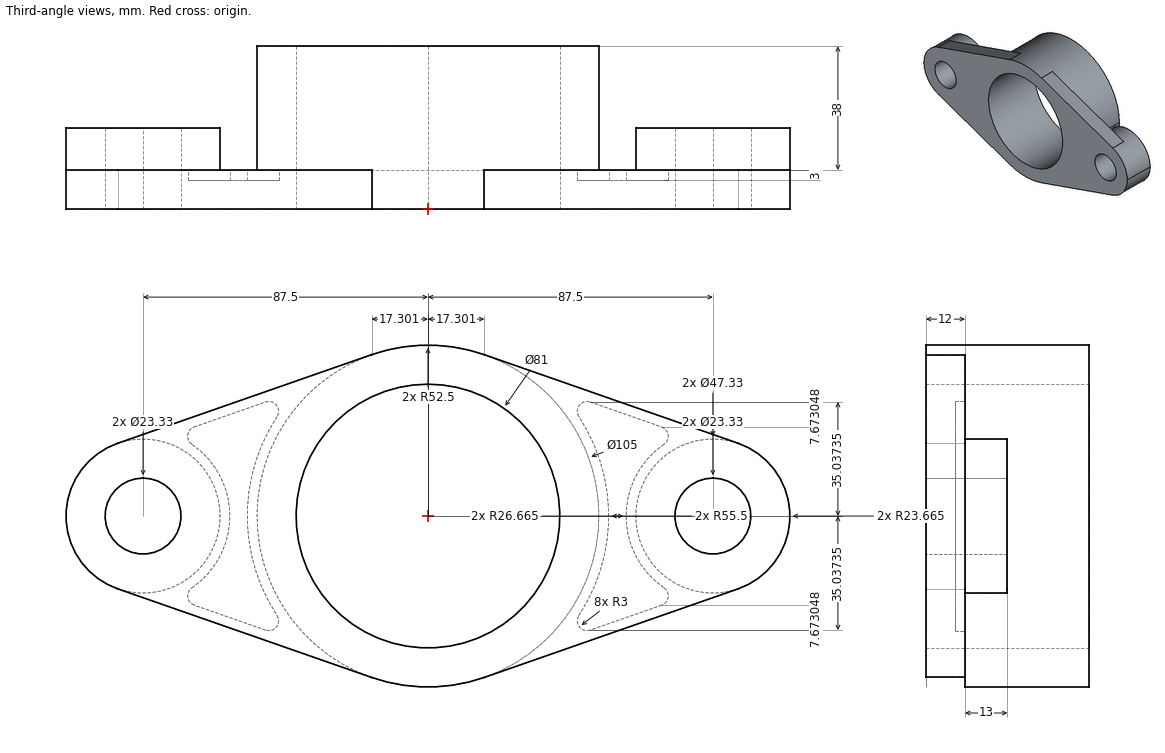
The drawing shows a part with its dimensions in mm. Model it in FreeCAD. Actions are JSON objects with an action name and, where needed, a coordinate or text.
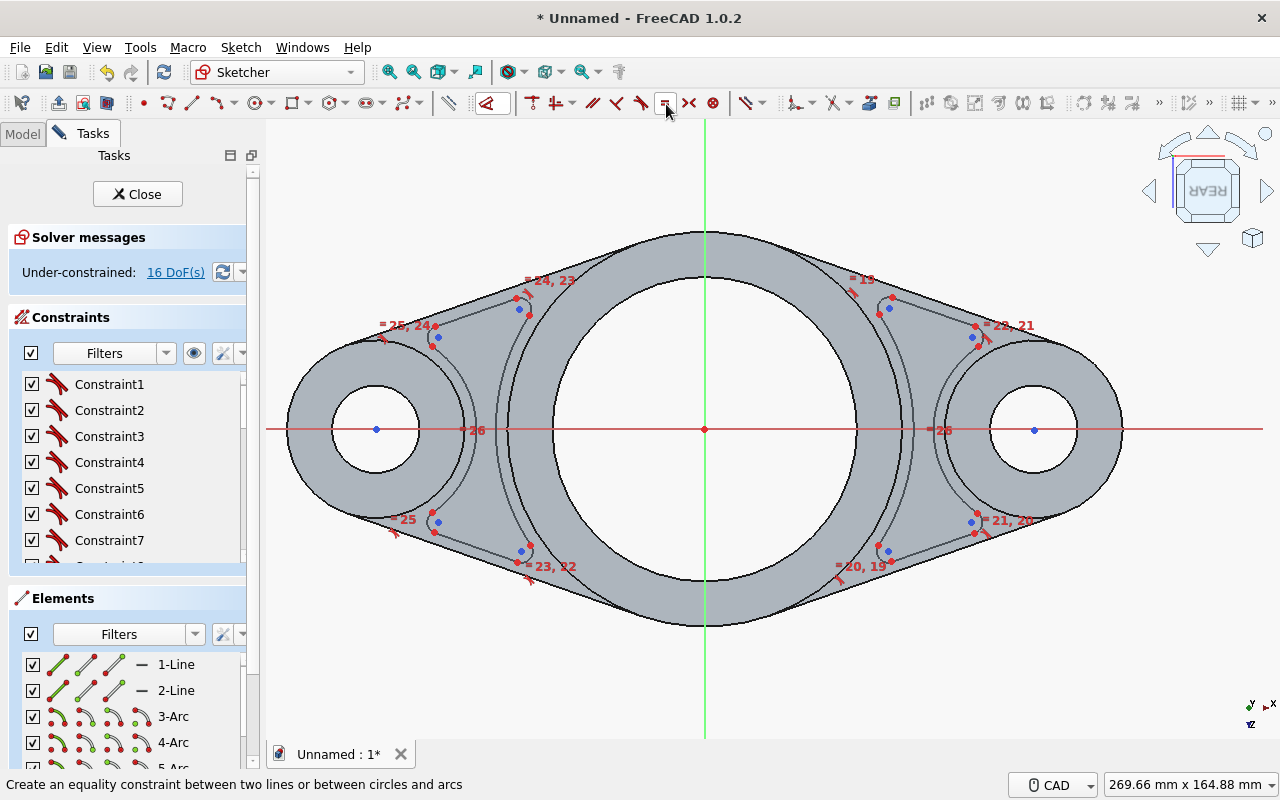
{"action": "left_click", "coordinate": [941, 391]}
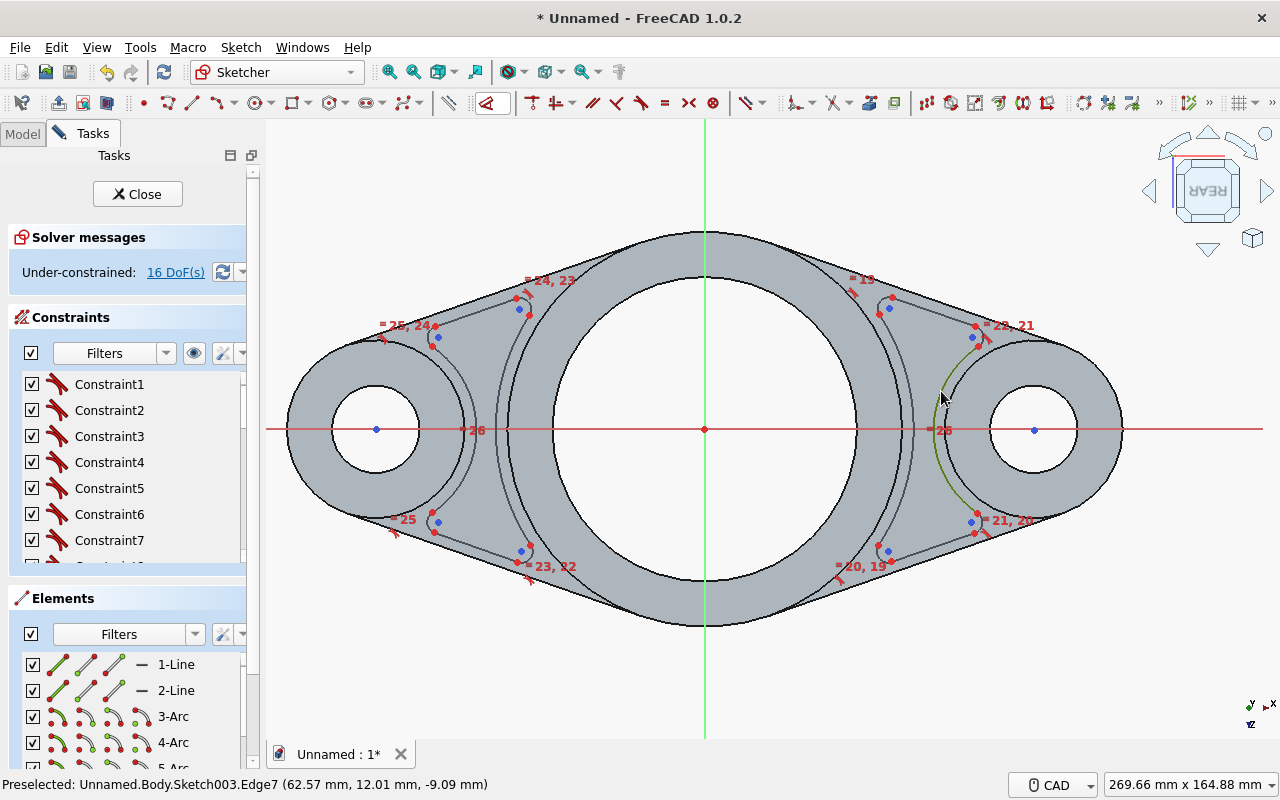
{"action": "left_click", "coordinate": [469, 468]}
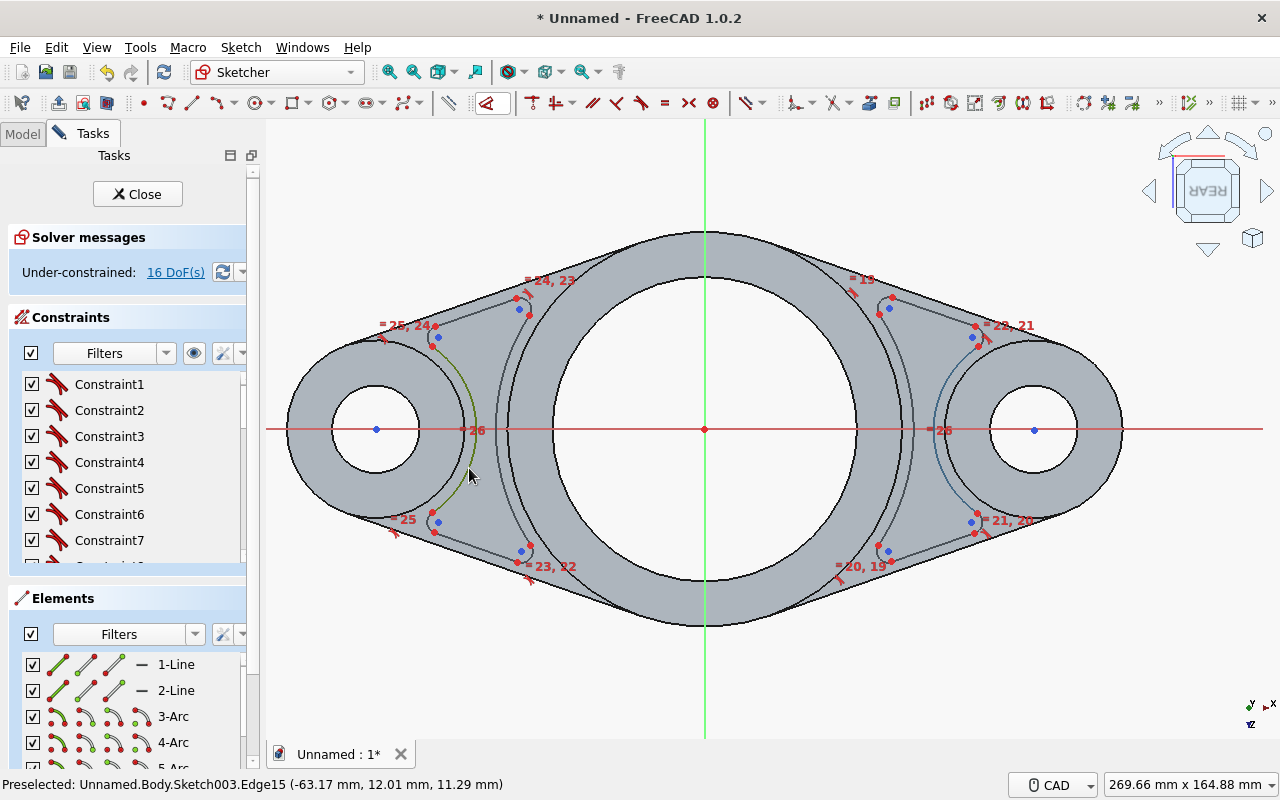
{"action": "left_click", "coordinate": [666, 104]}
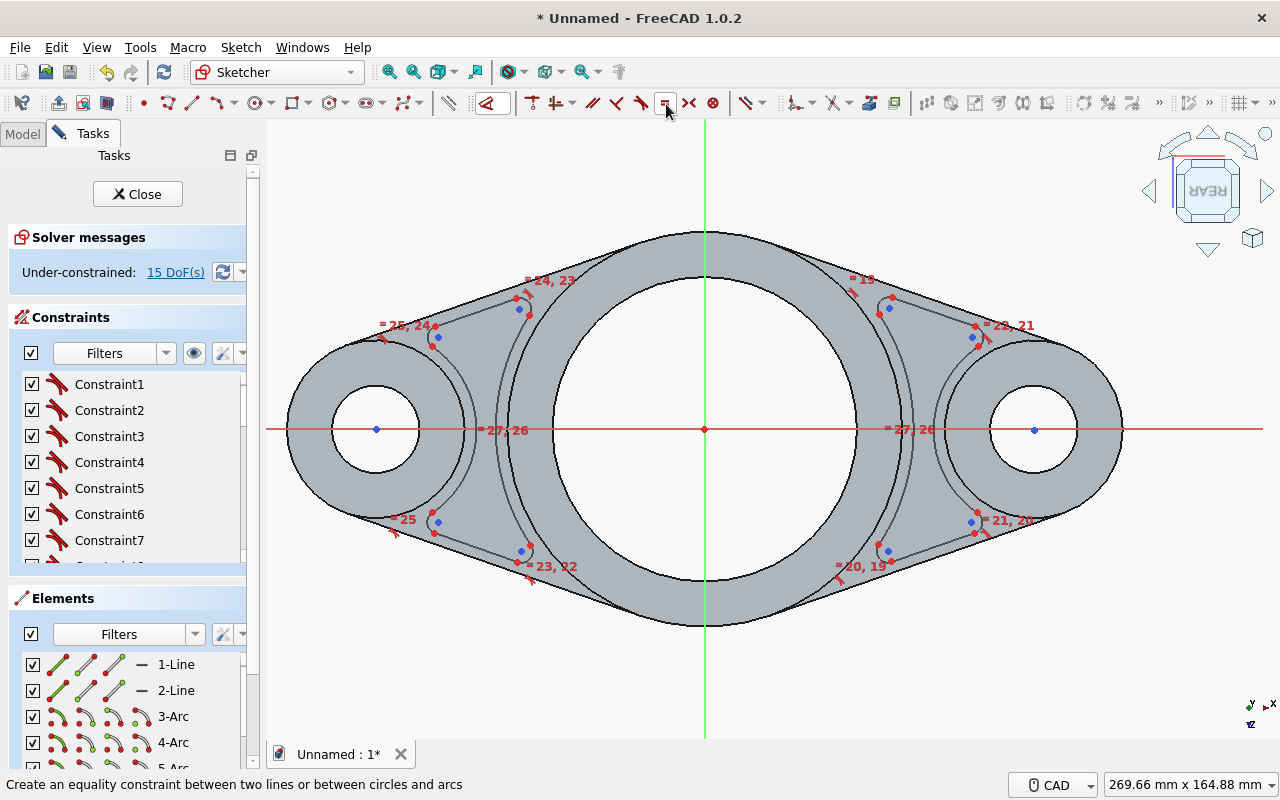
{"action": "left_click", "coordinate": [1034, 430]}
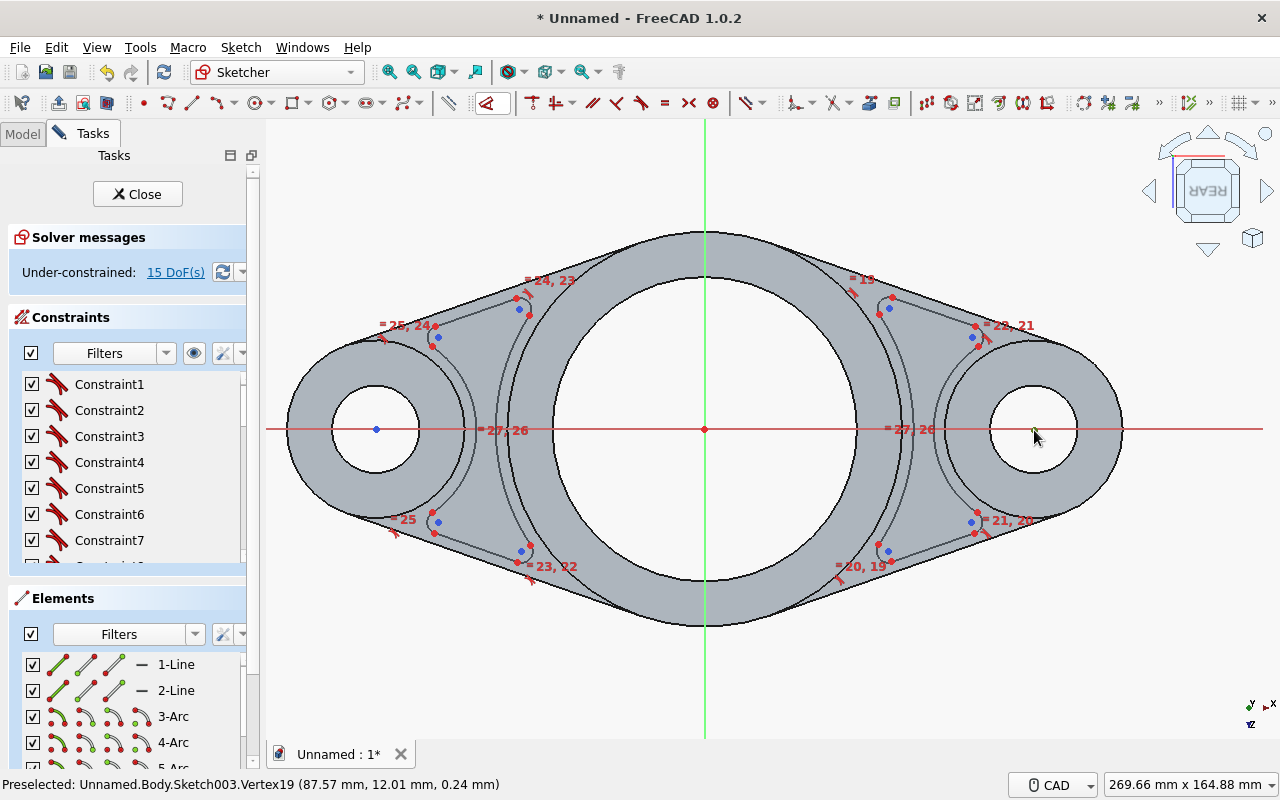
{"action": "left_click", "coordinate": [353, 429]}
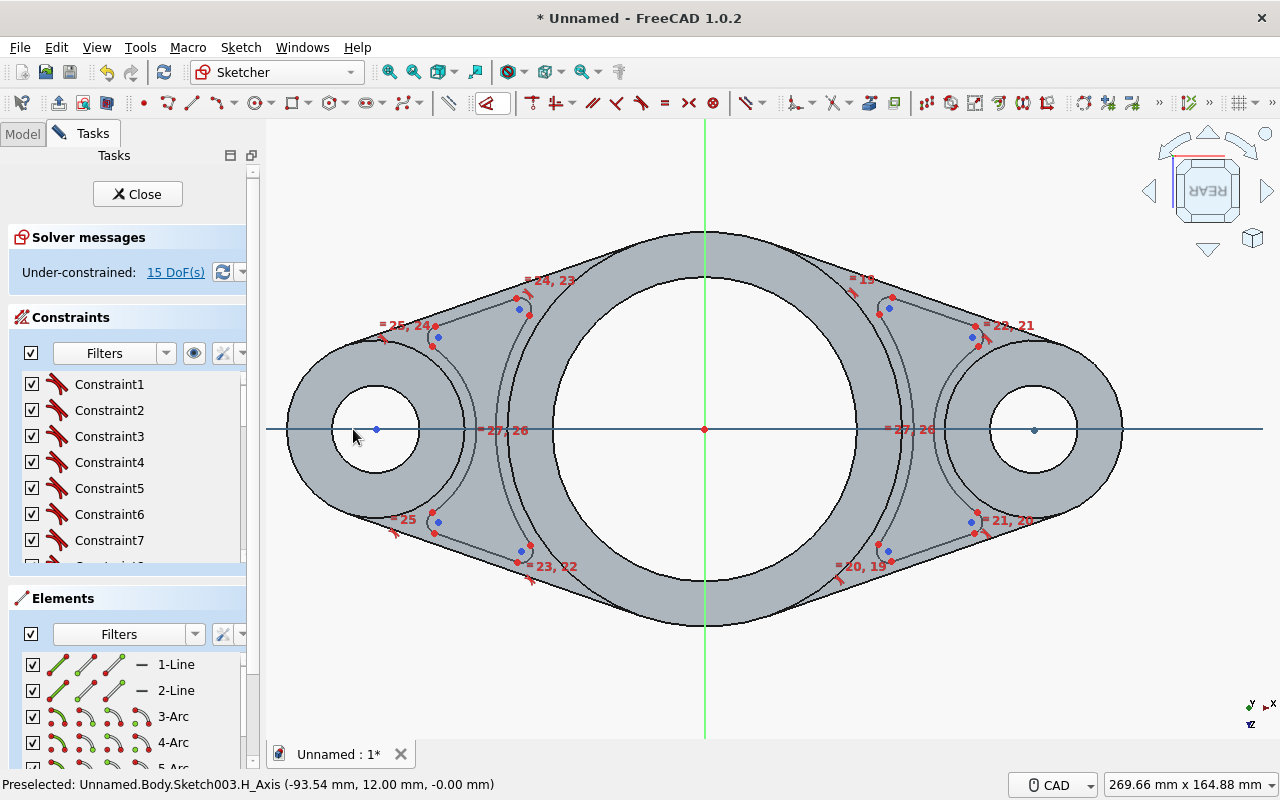
{"action": "left_click", "coordinate": [532, 104]}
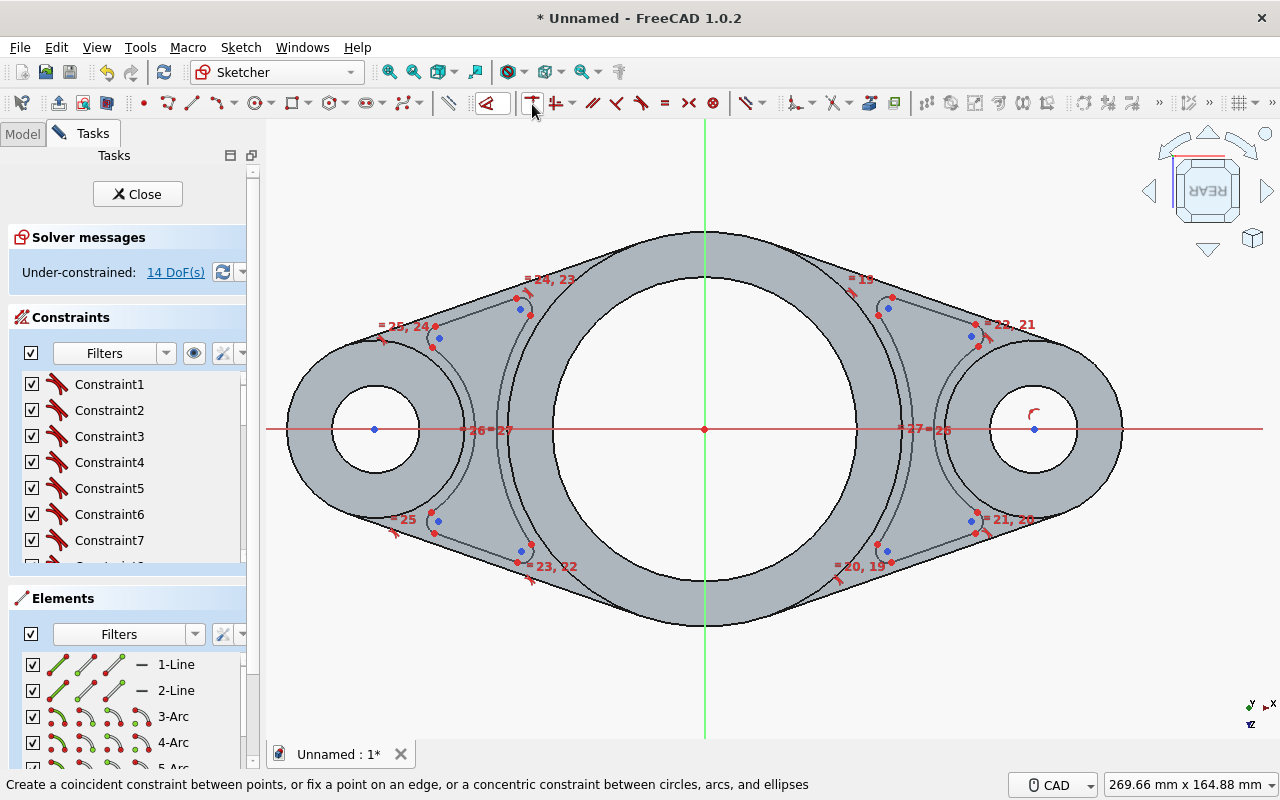
{"action": "left_click", "coordinate": [375, 430]}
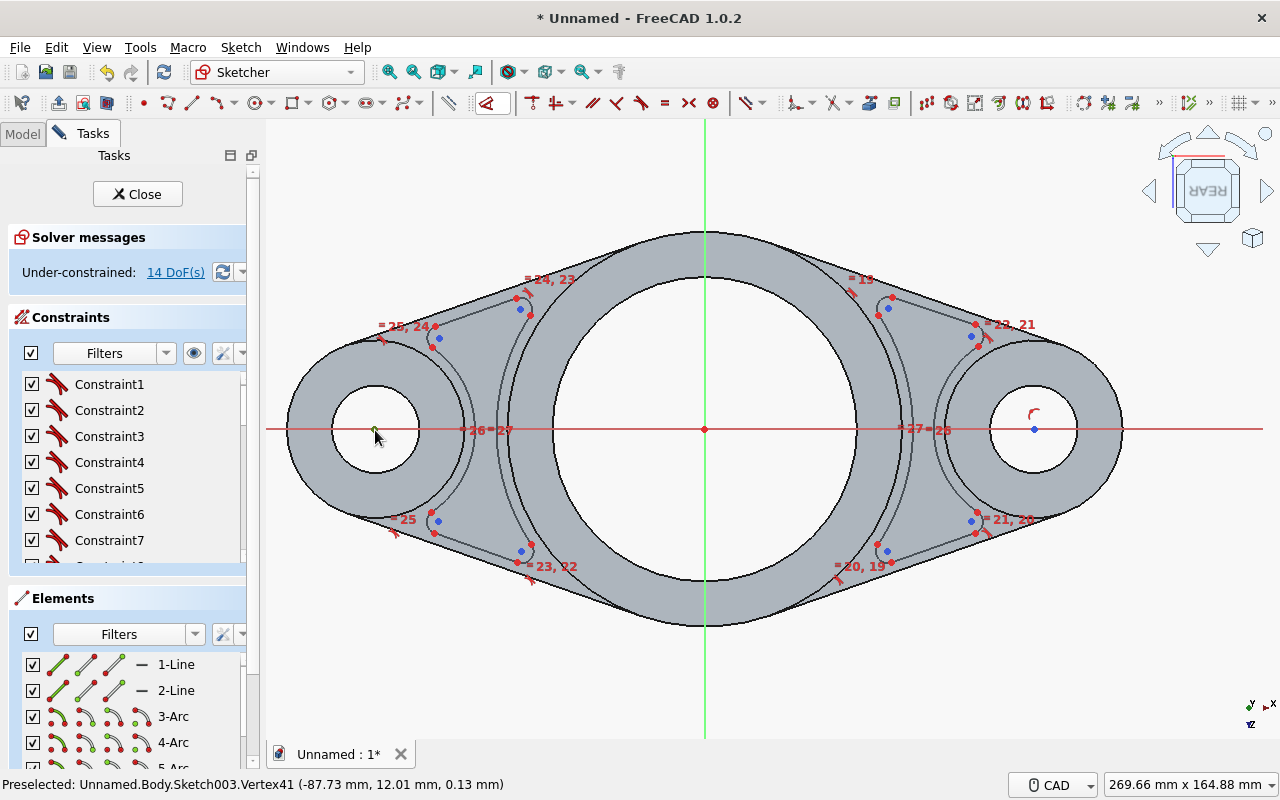
{"action": "left_click", "coordinate": [353, 429]}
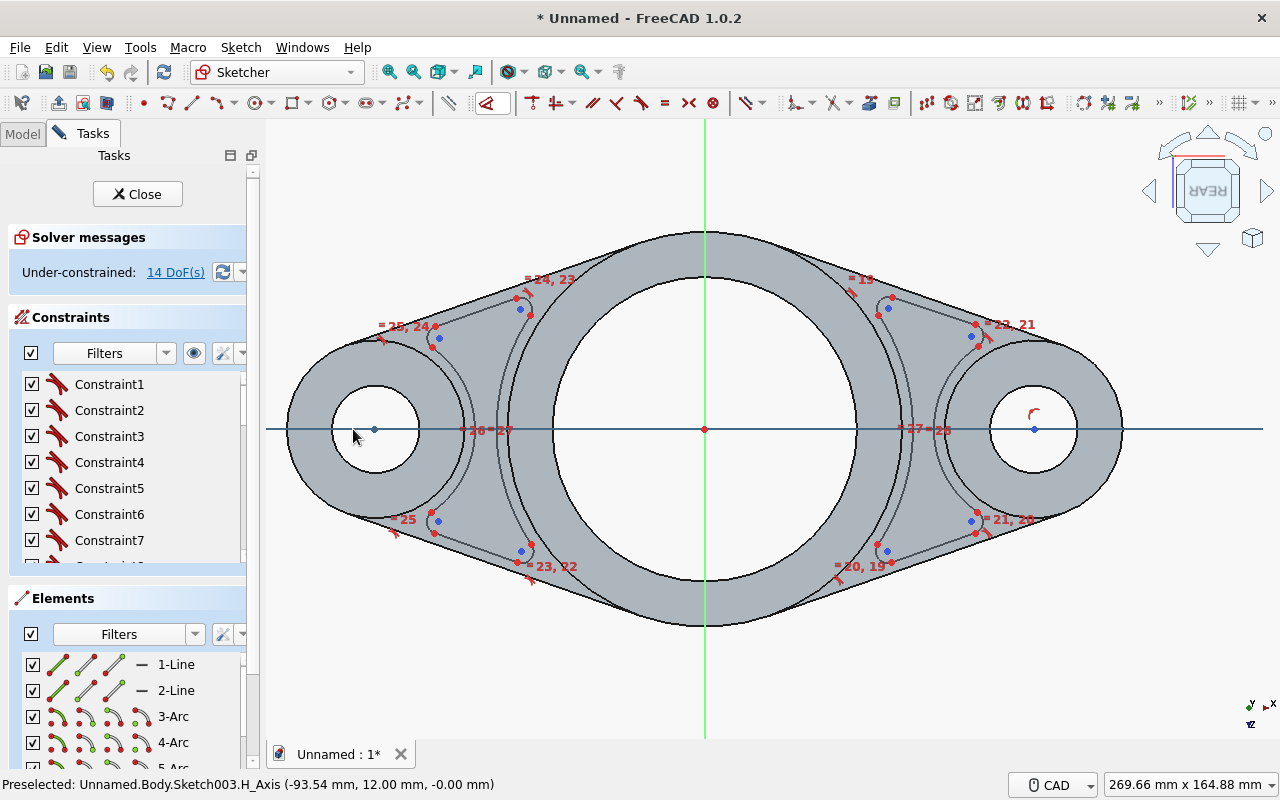
{"action": "left_click", "coordinate": [532, 104]}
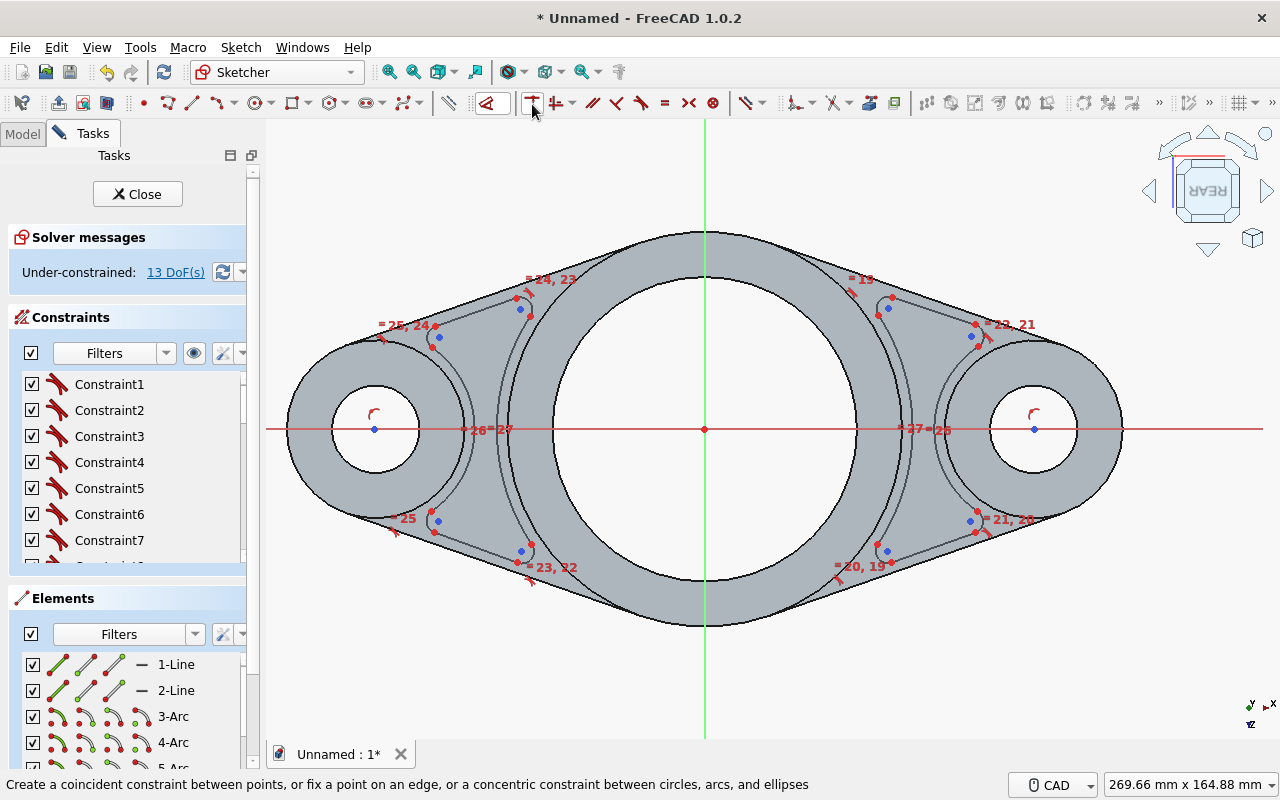
{"action": "scroll", "coordinate": [879, 301], "scroll_direction": "up", "scroll_amount": 7}